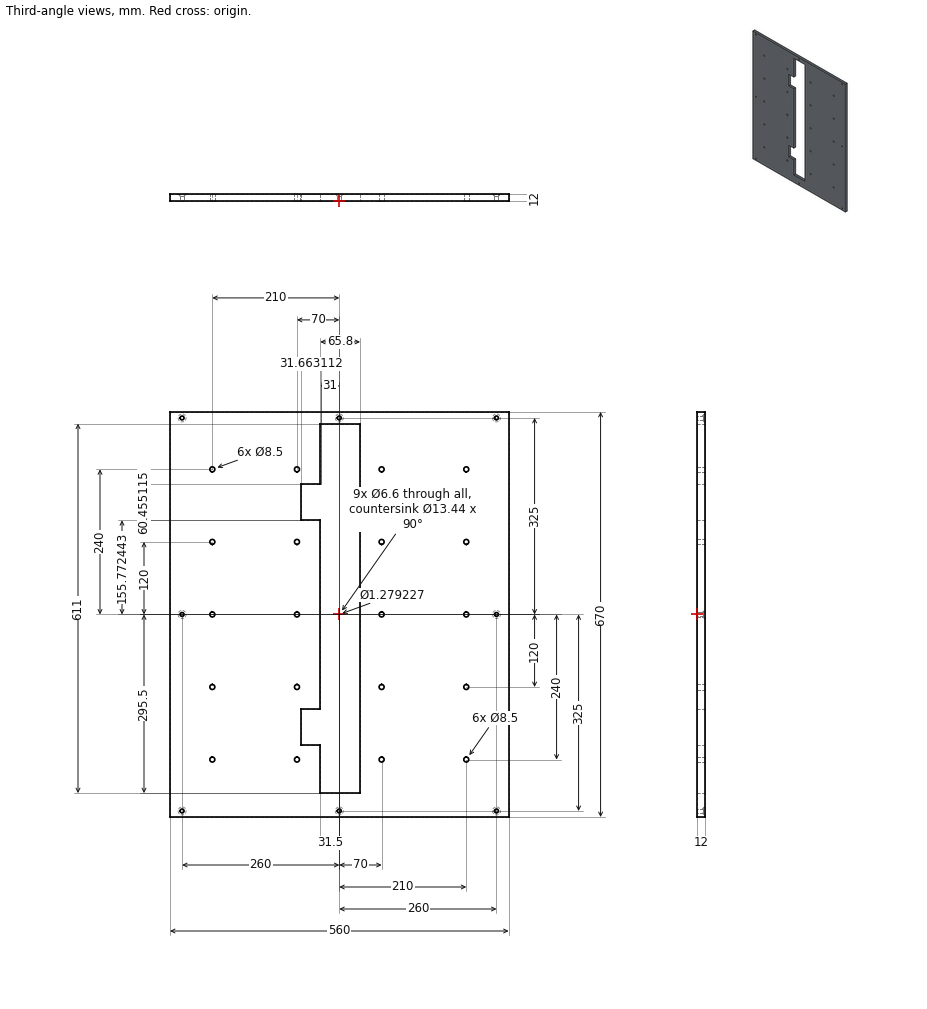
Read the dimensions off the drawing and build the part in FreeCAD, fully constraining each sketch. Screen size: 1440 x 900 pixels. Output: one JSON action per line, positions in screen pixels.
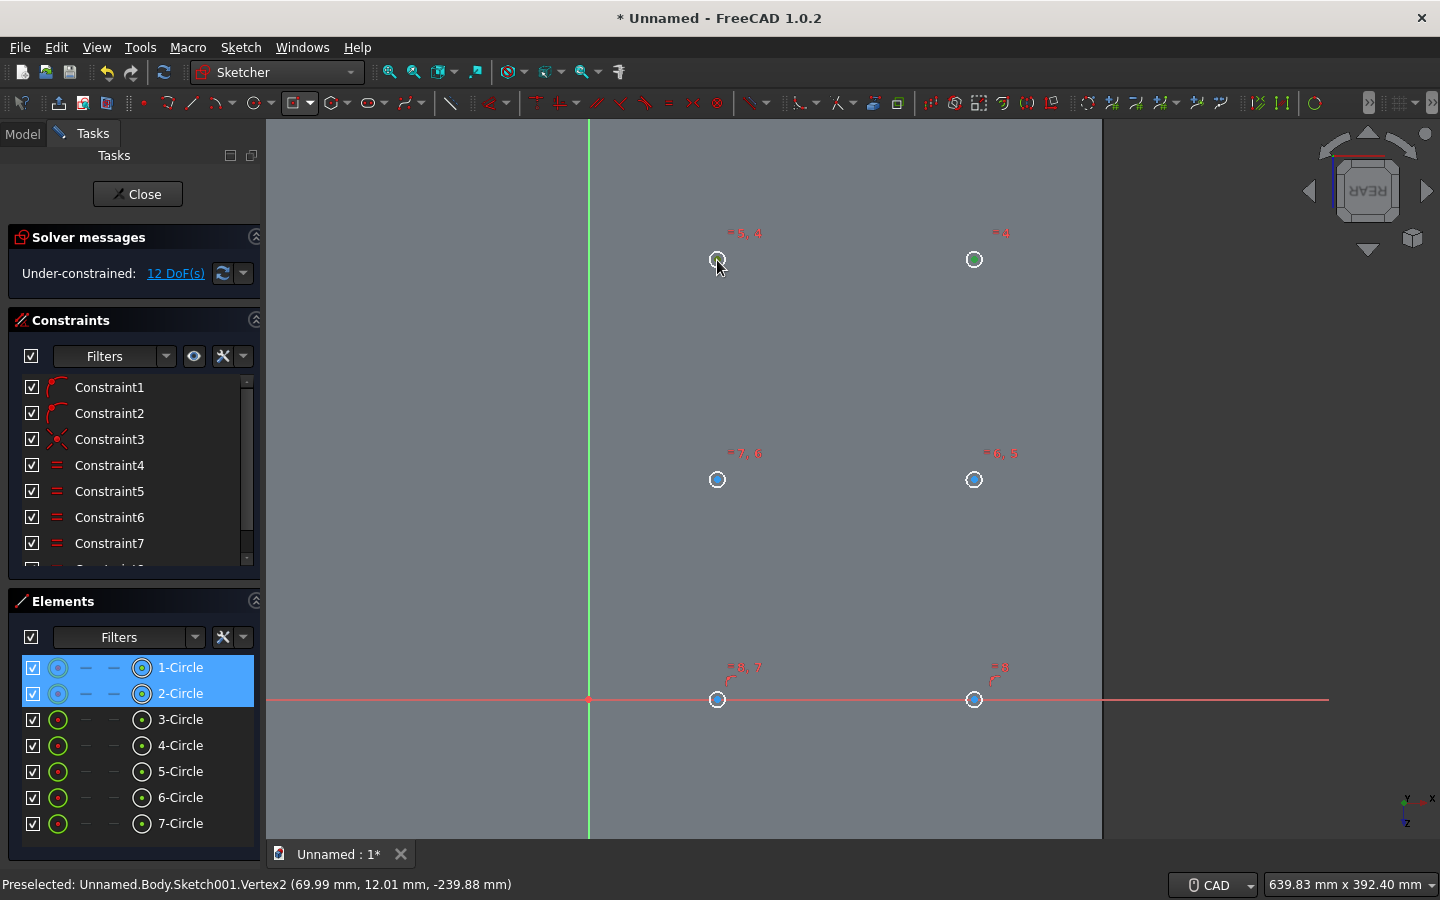
{"action": "key", "text": "h"}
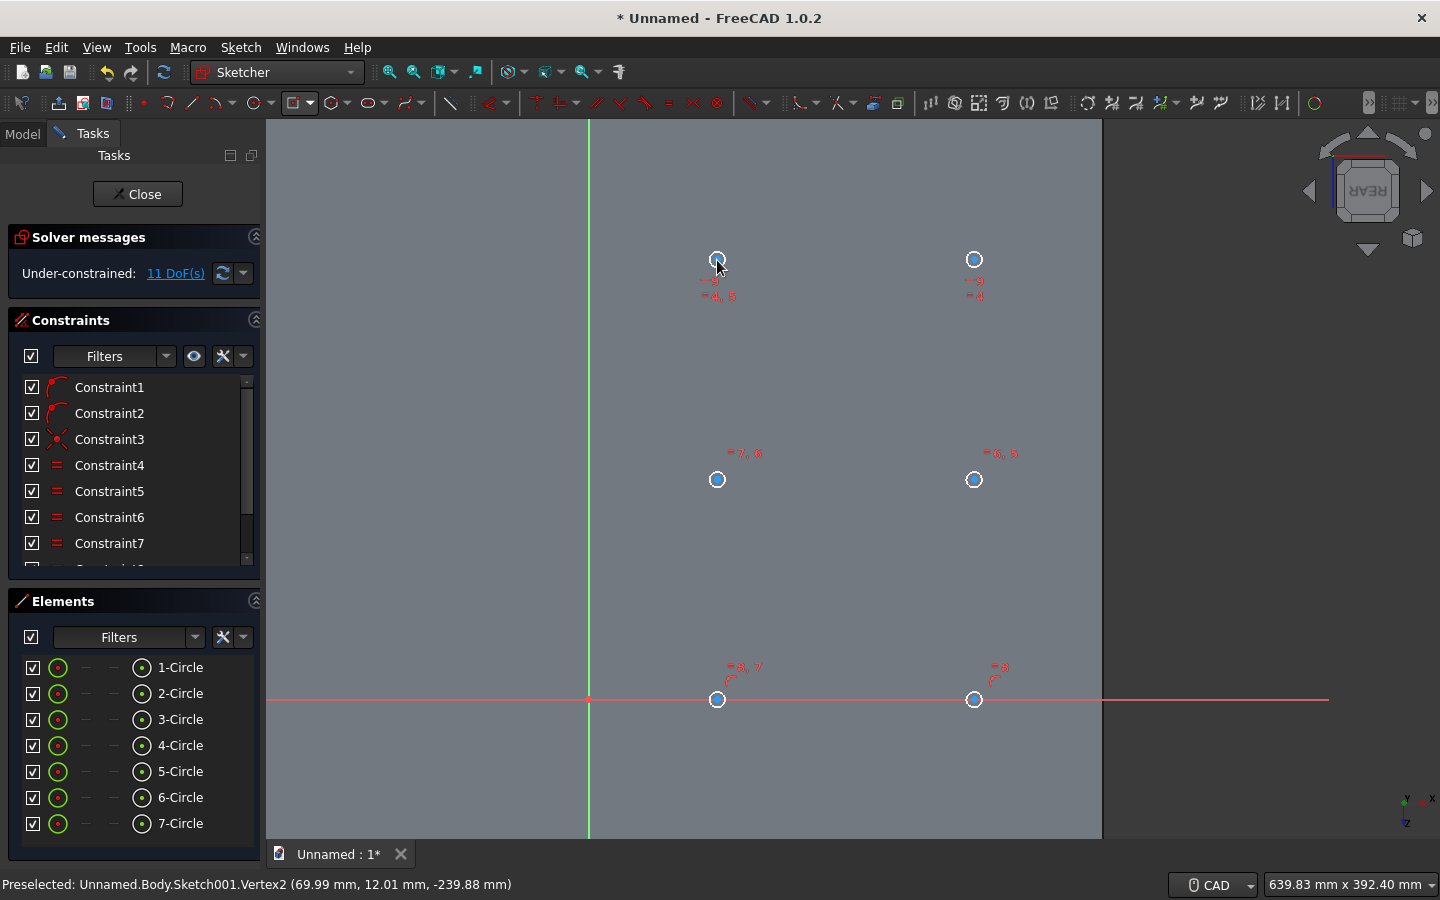
{"action": "left_click", "coordinate": [974, 260]}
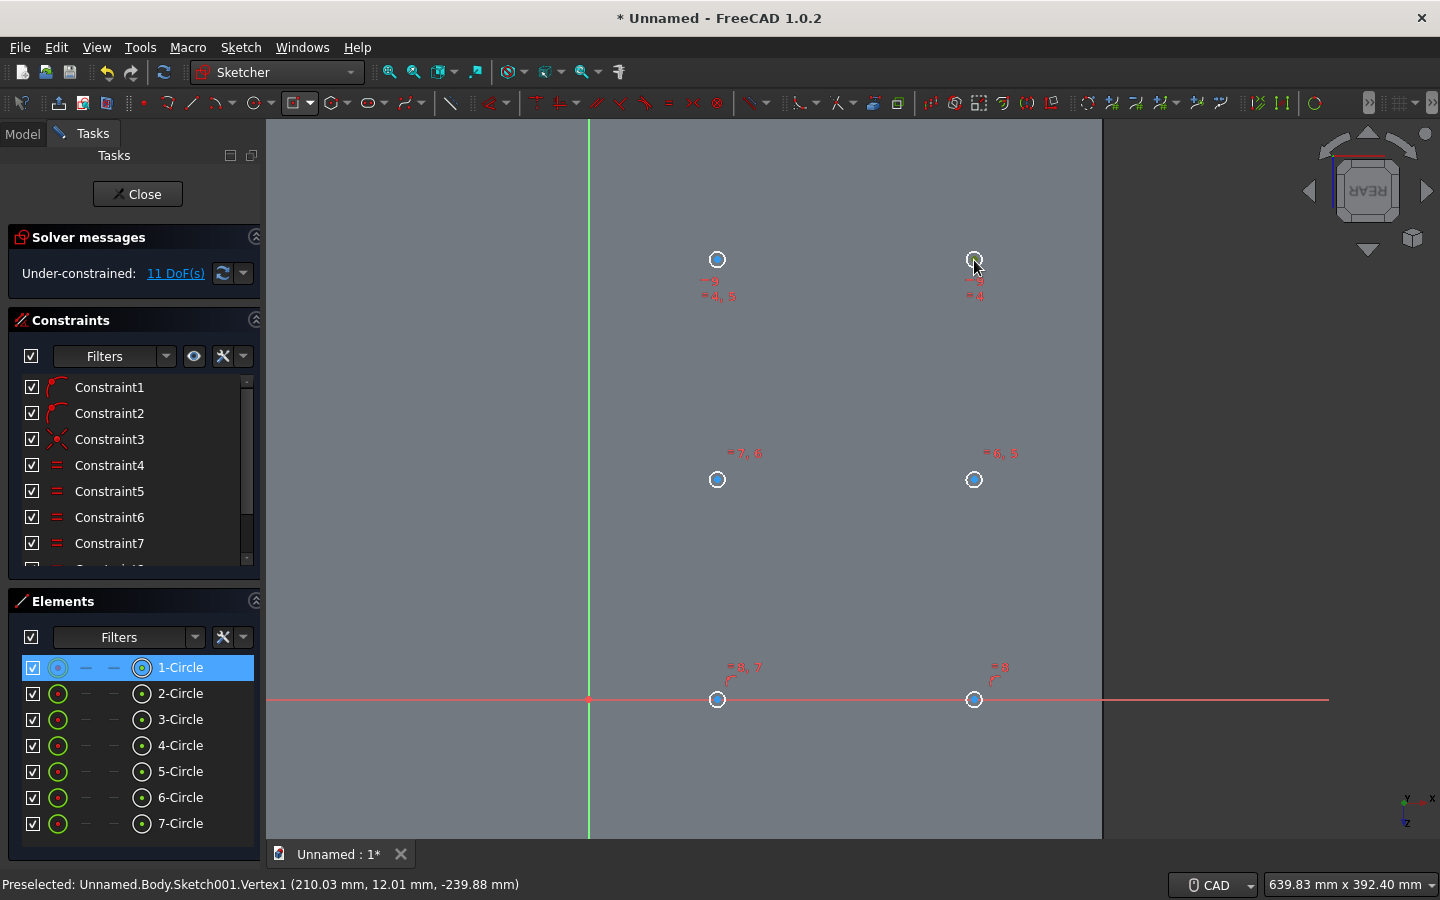
{"action": "left_click", "coordinate": [974, 480]}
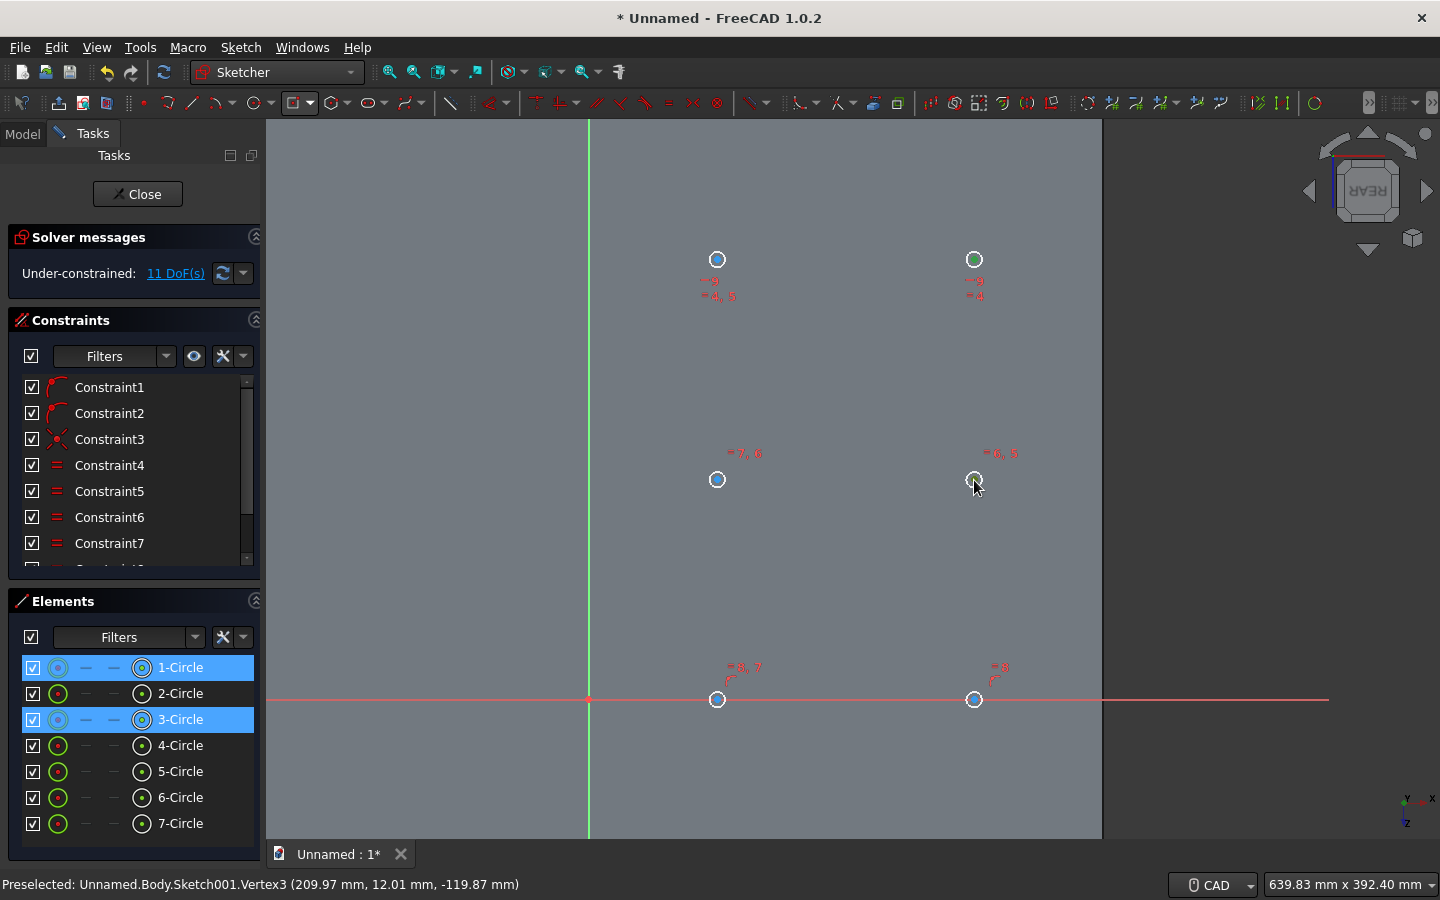
{"action": "left_click", "coordinate": [578, 104]}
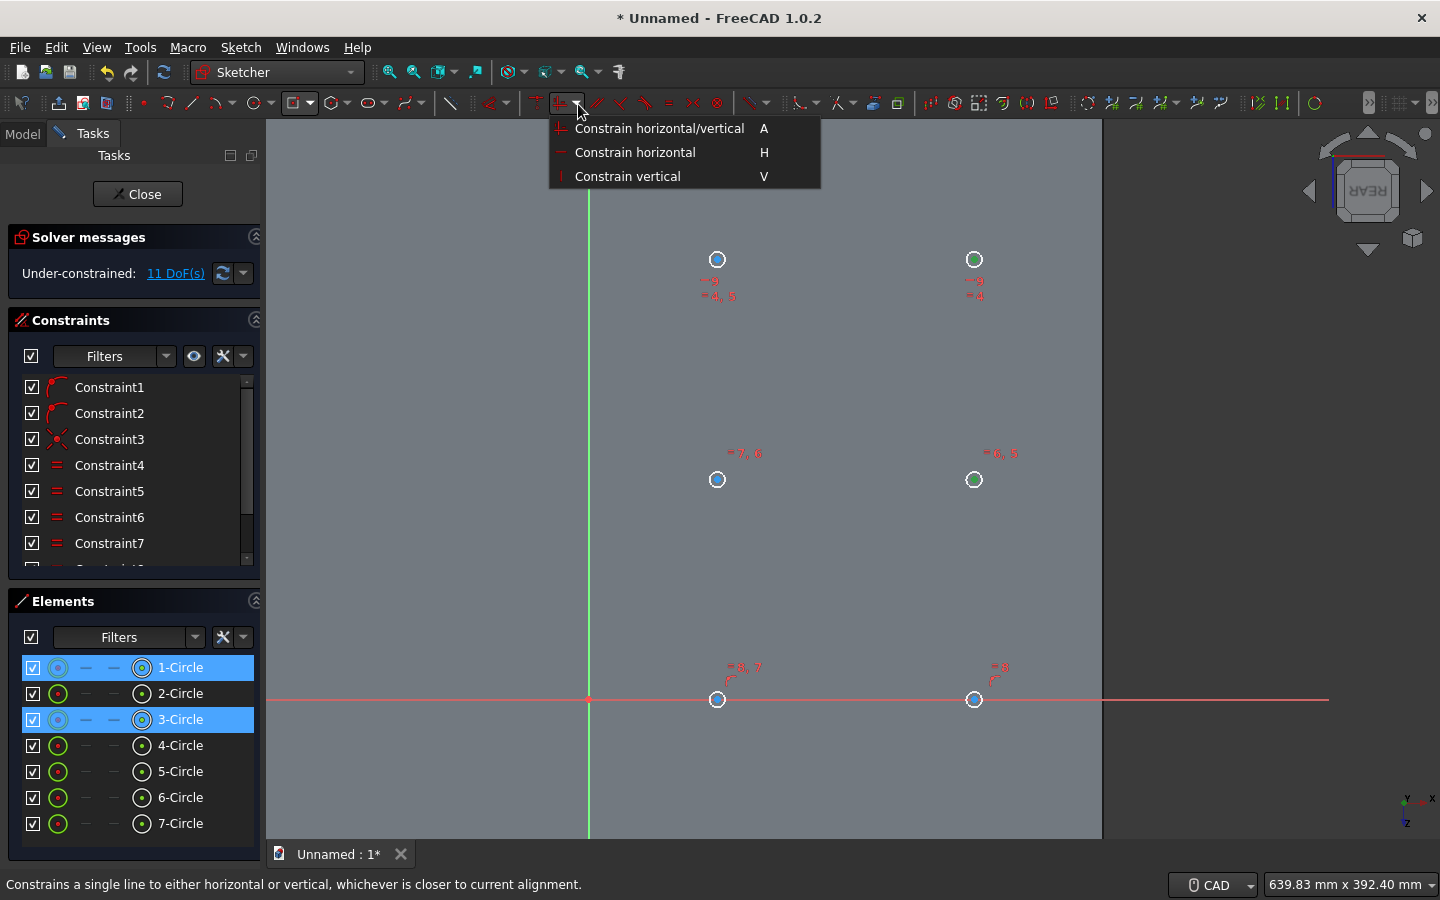
{"action": "left_click", "coordinate": [685, 176]}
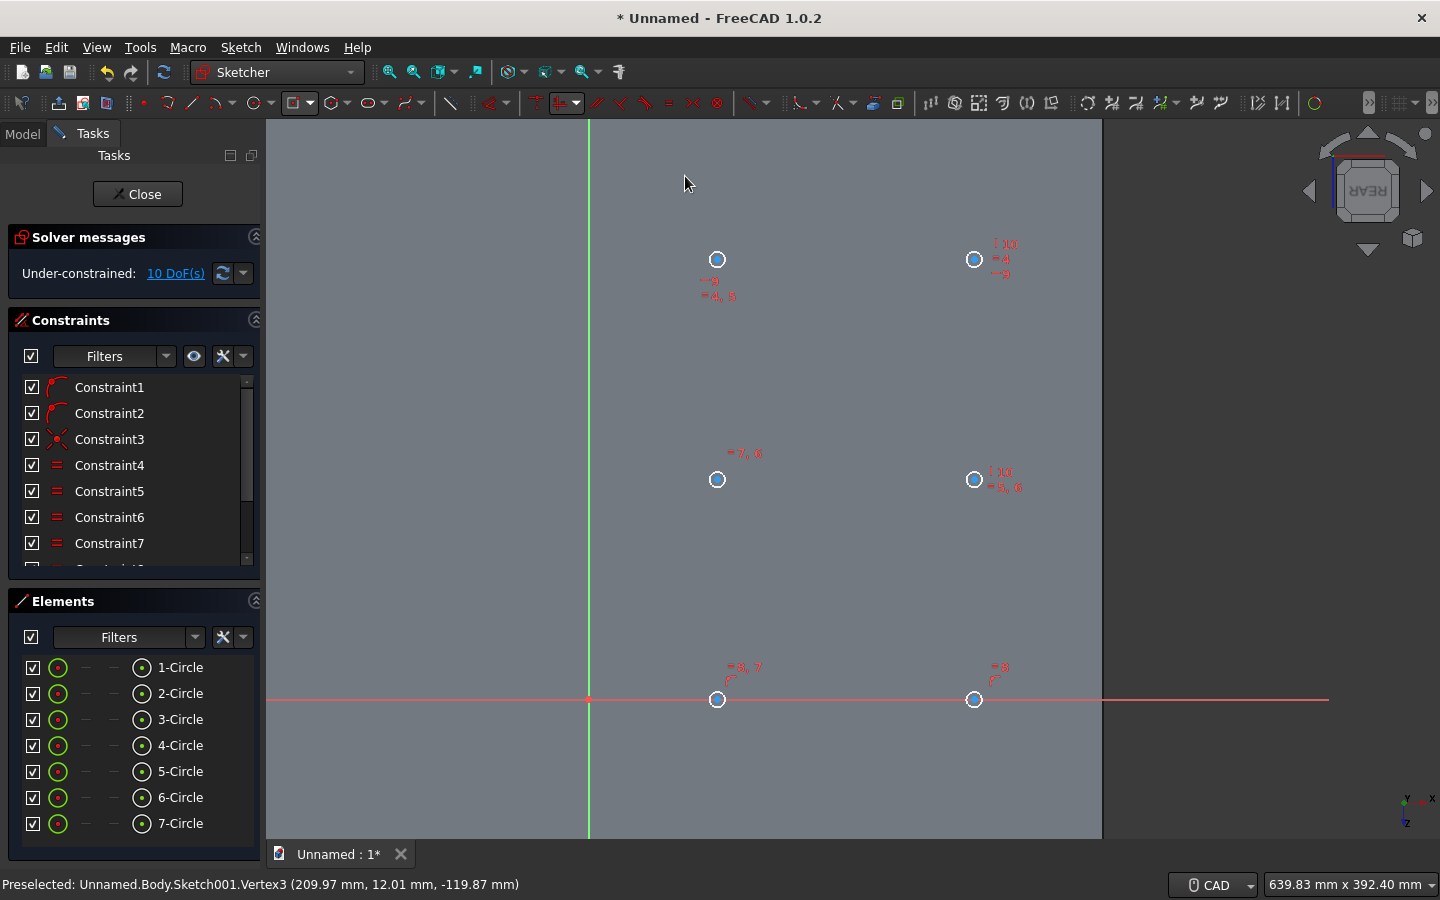
{"action": "left_click", "coordinate": [717, 260]}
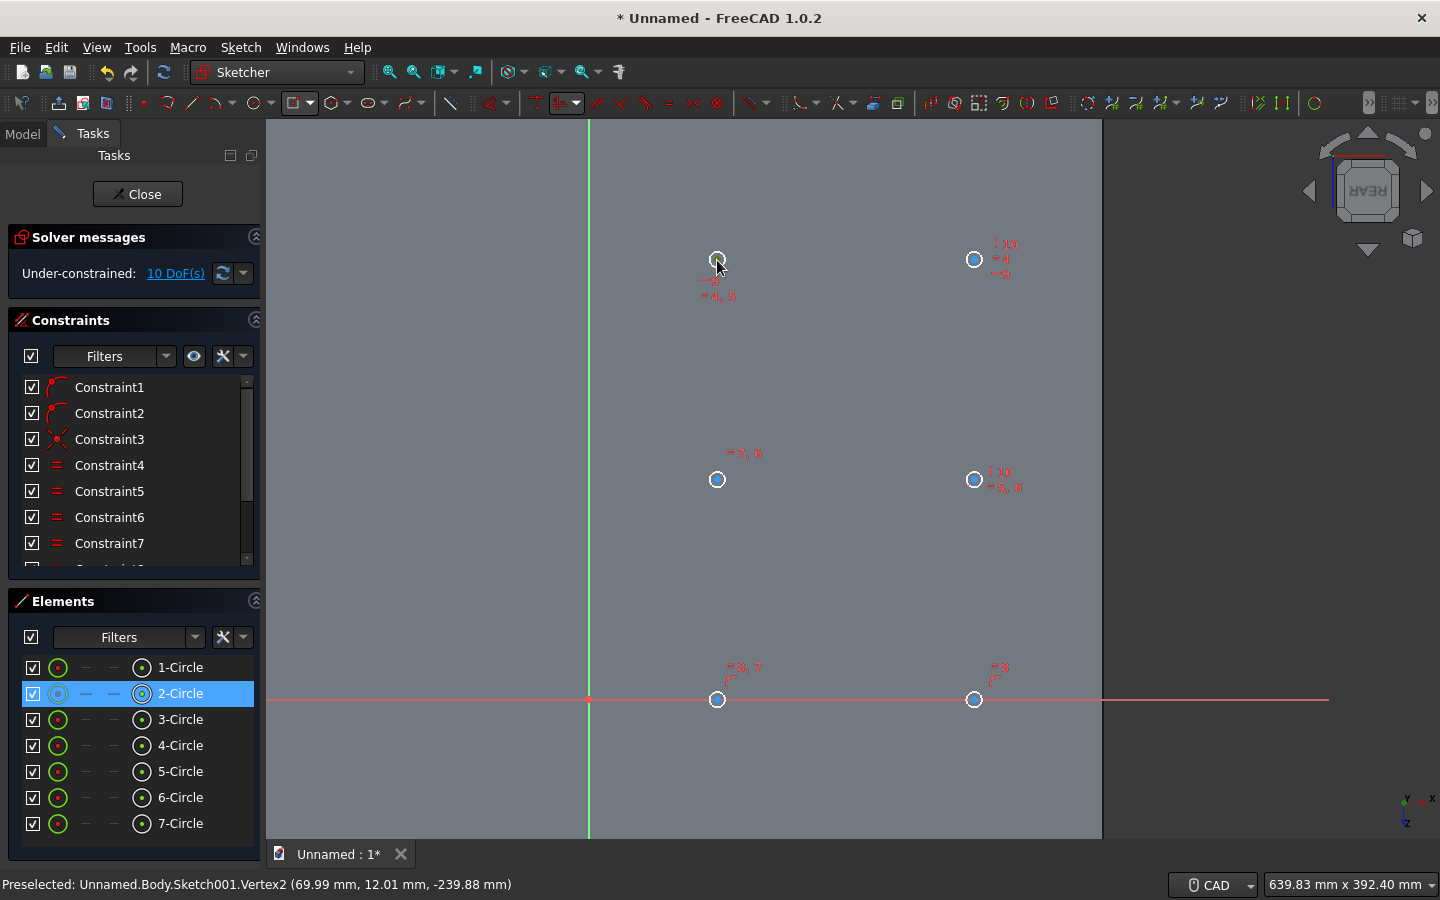
{"action": "left_click", "coordinate": [717, 480]}